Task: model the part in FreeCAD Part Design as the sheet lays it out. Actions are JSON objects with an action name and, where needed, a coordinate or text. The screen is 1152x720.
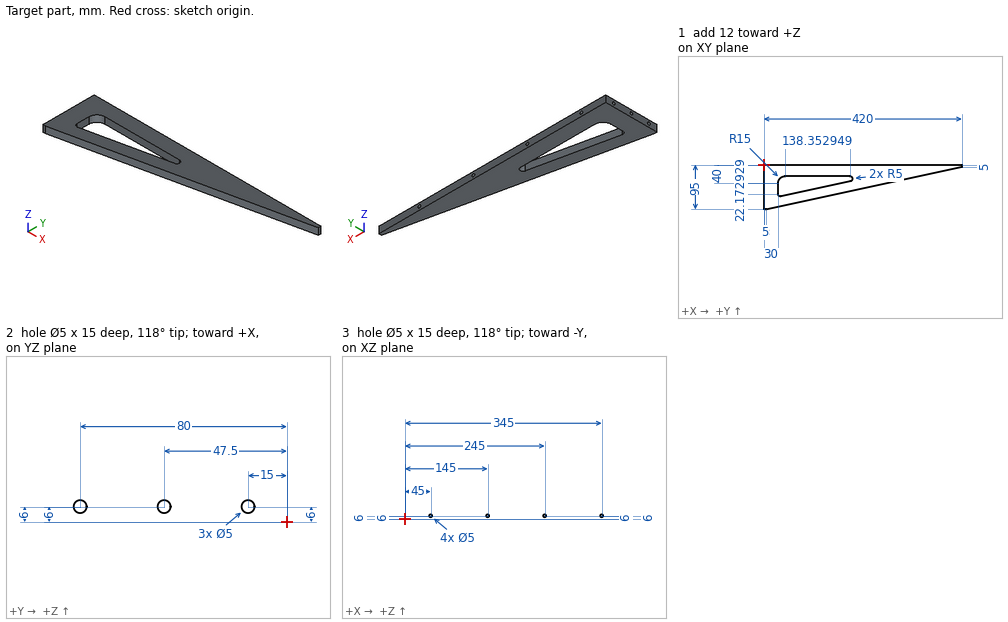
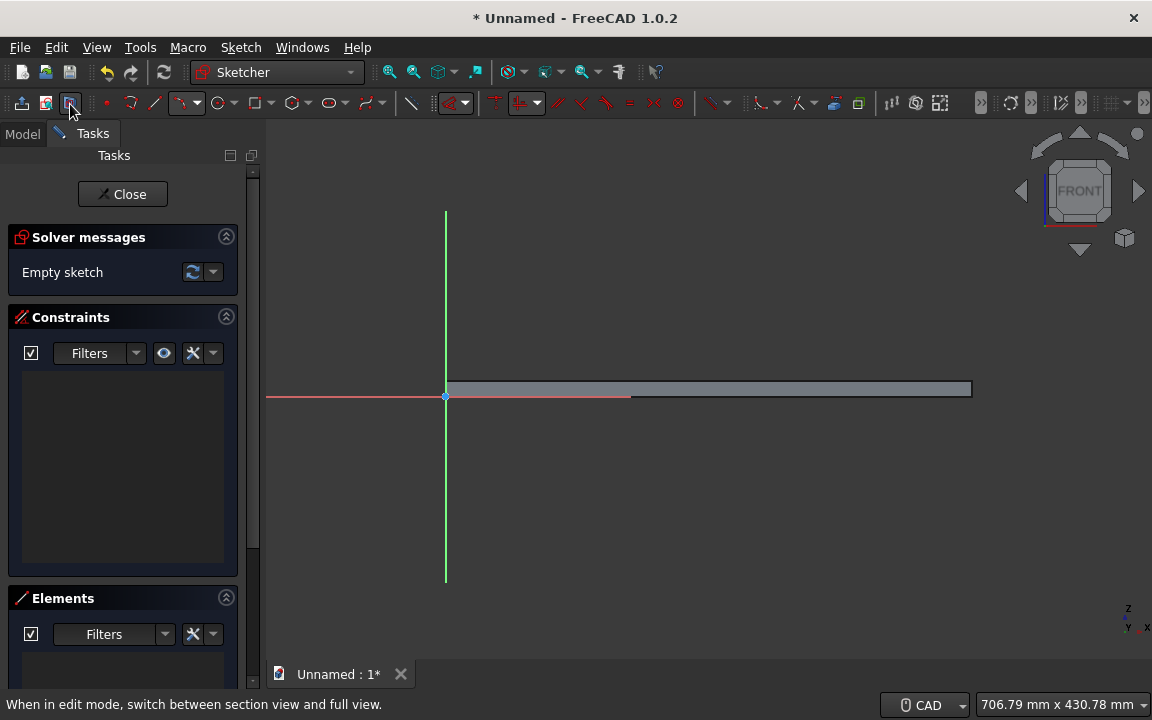
{"action": "left_click", "coordinate": [218, 104]}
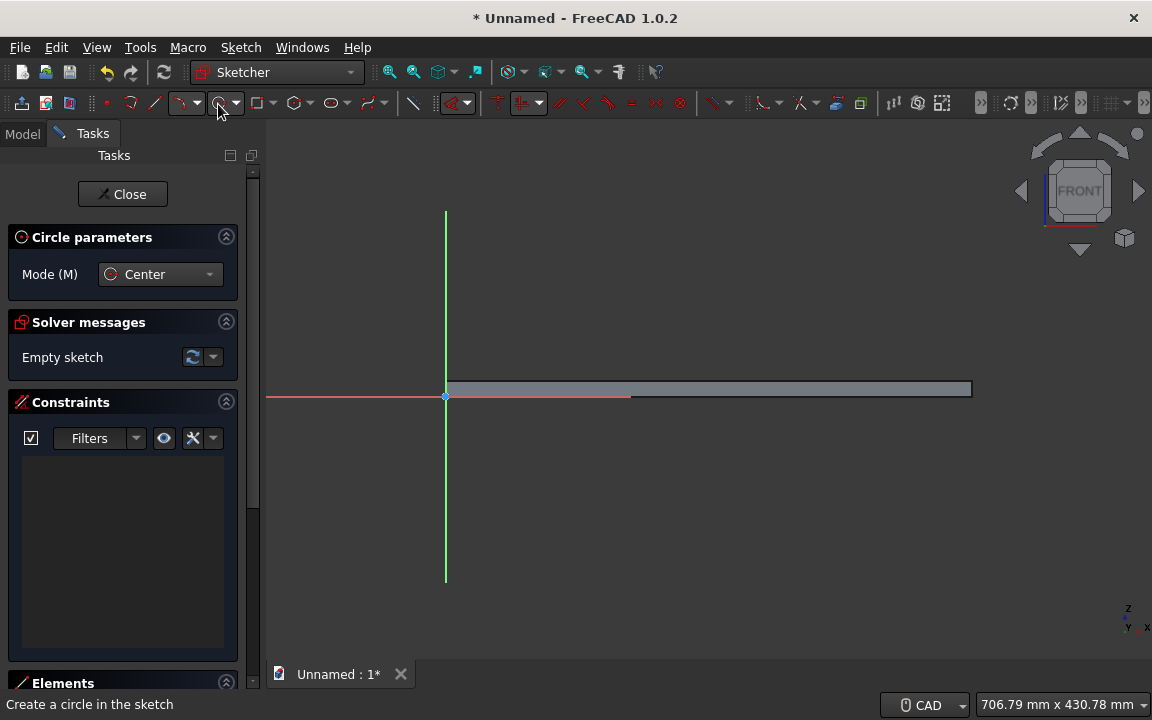
{"action": "scroll", "coordinate": [502, 389], "scroll_direction": "up", "scroll_amount": 10}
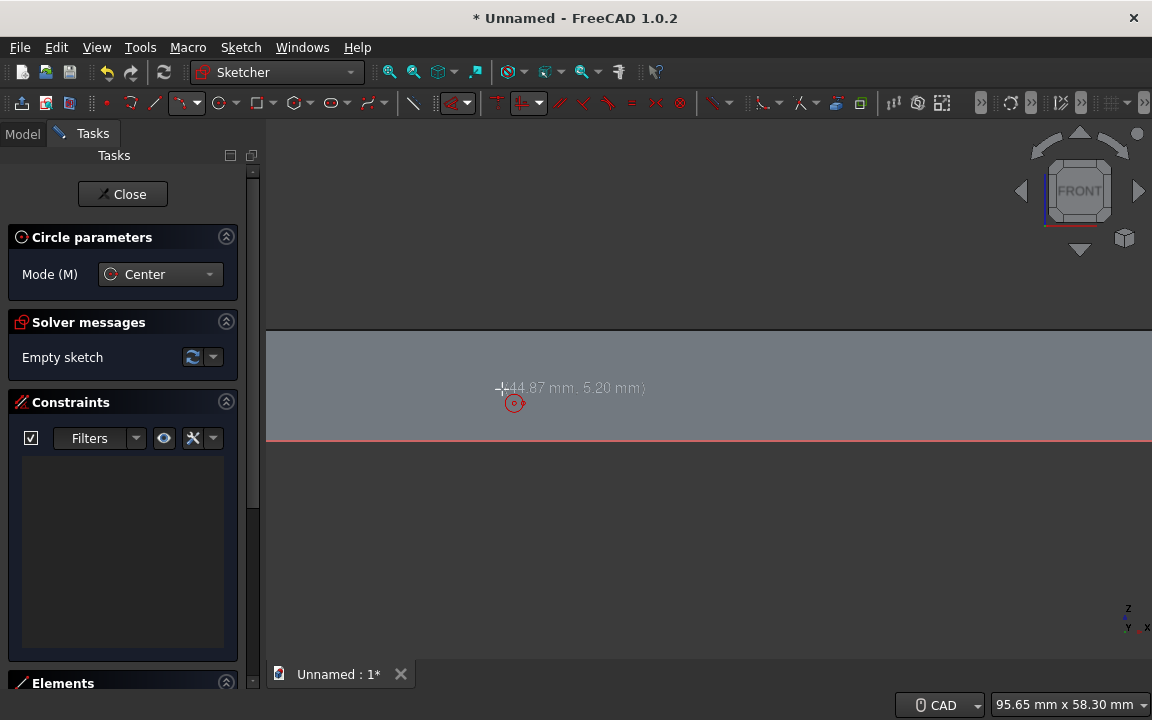
{"action": "scroll", "coordinate": [432, 386], "scroll_direction": "down", "scroll_amount": 9}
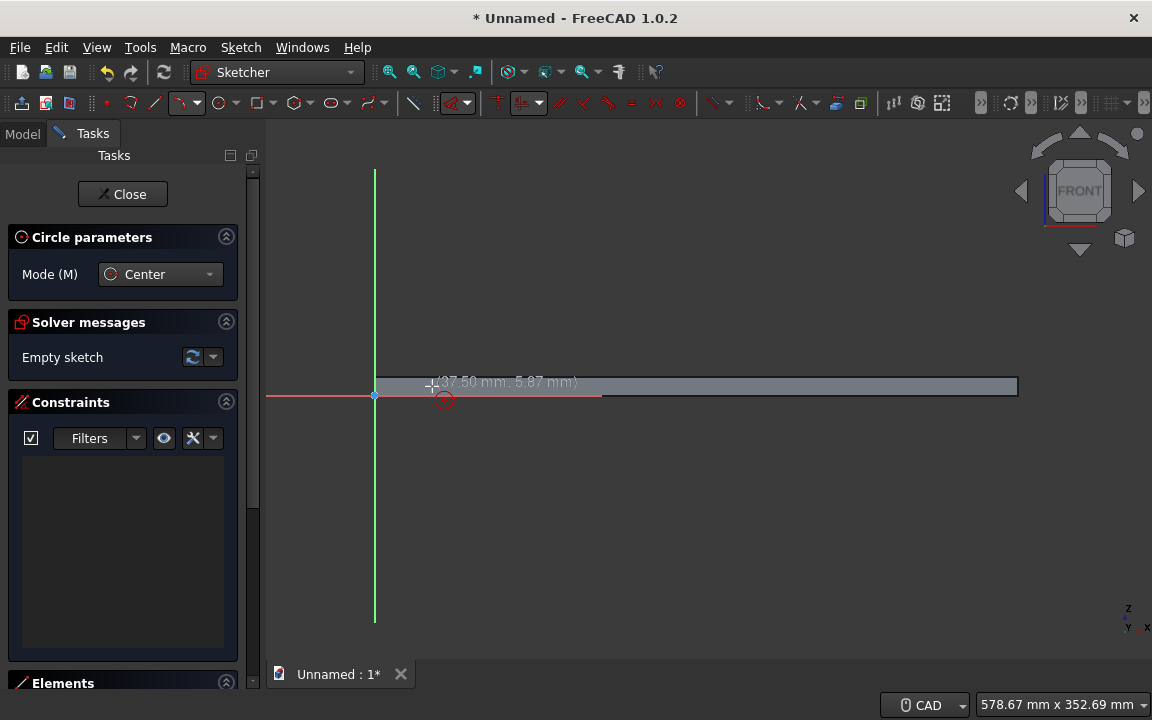
{"action": "scroll", "coordinate": [444, 386], "scroll_direction": "up", "scroll_amount": 3}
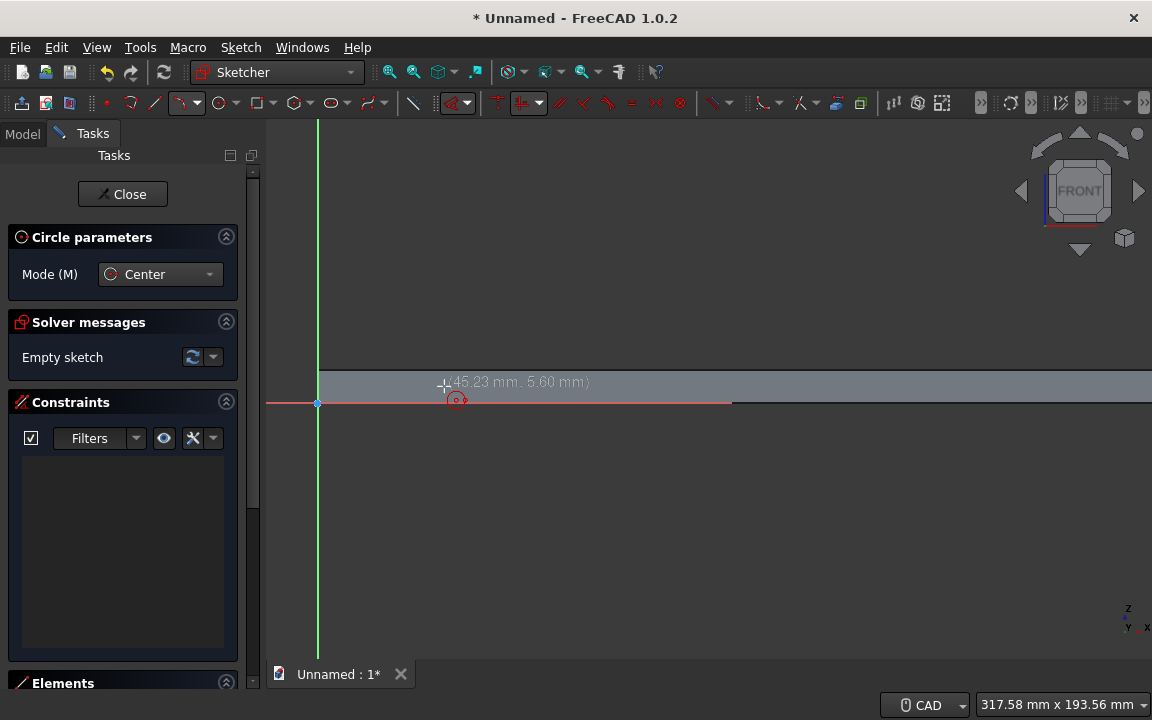
{"action": "left_click", "coordinate": [443, 386]}
{"action": "mouse_move", "coordinate": [448, 381]}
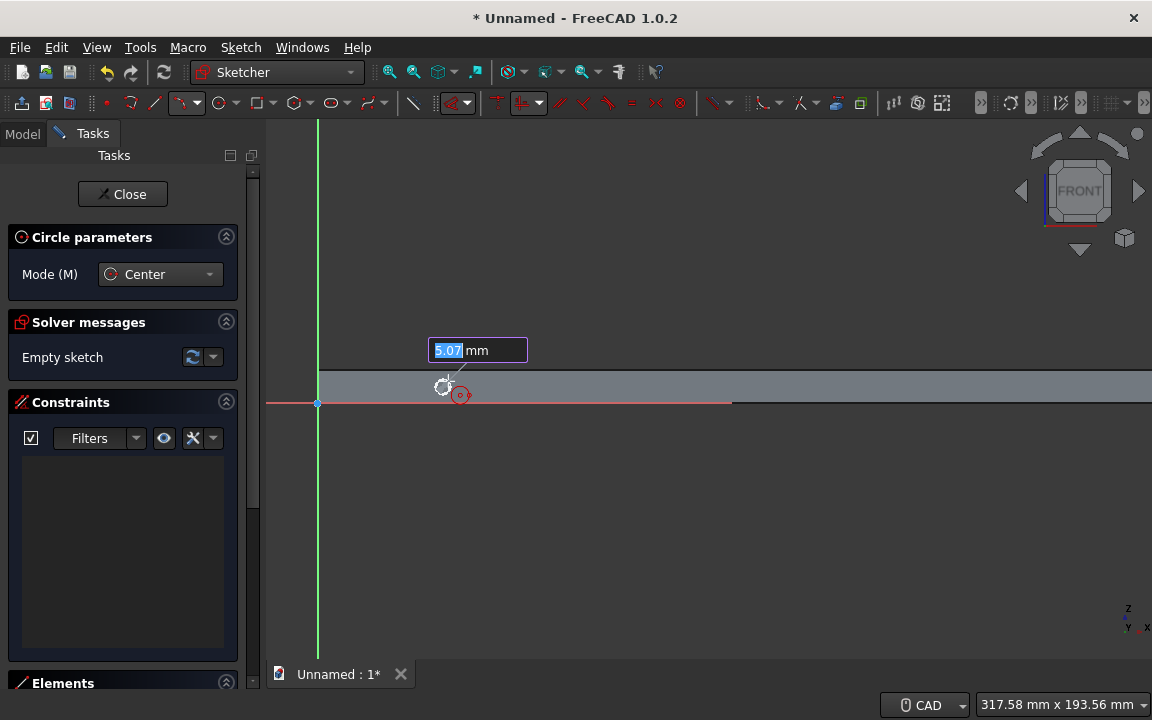
{"action": "type", "text": "5"}
{"action": "key", "text": "Return"}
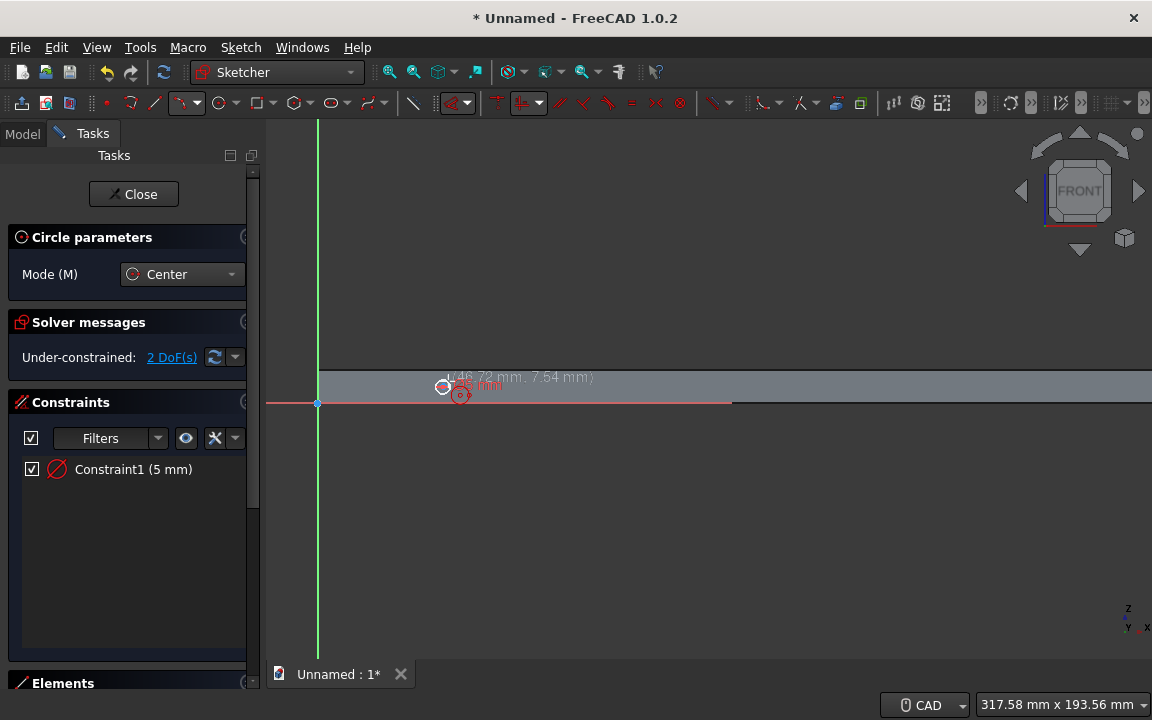
{"action": "scroll", "coordinate": [722, 386], "scroll_direction": "up", "scroll_amount": 6}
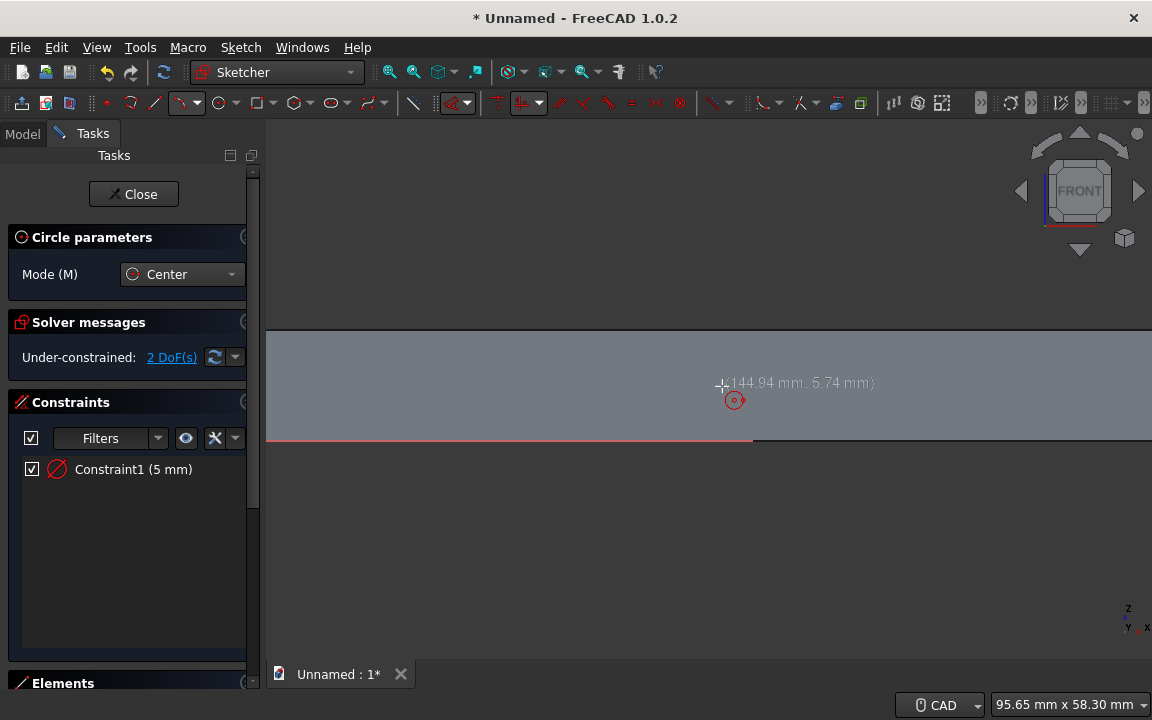
{"action": "scroll", "coordinate": [572, 386], "scroll_direction": "down", "scroll_amount": 9}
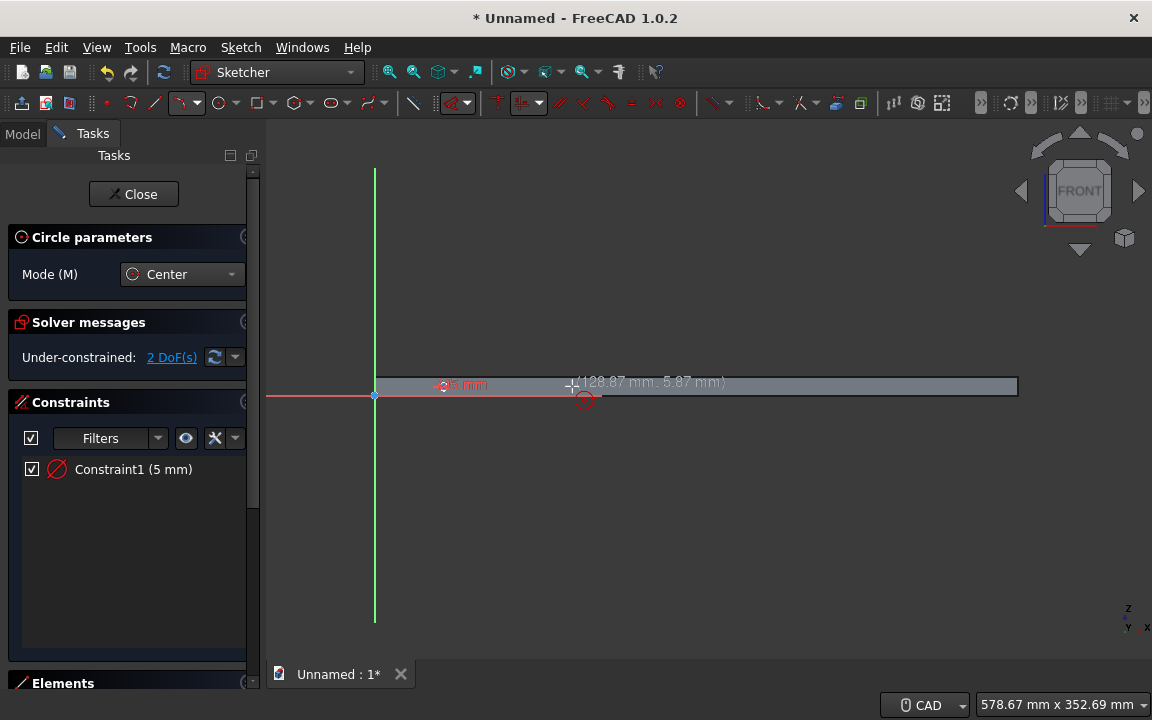
{"action": "scroll", "coordinate": [597, 386], "scroll_direction": "up", "scroll_amount": 3}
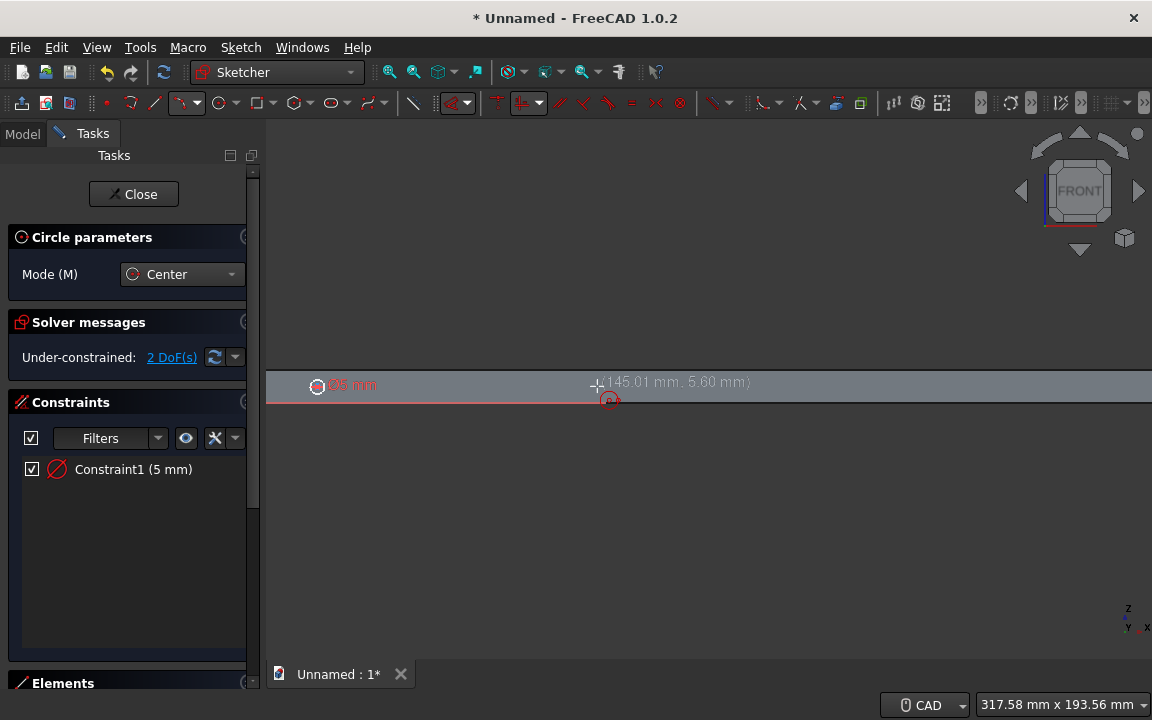
{"action": "left_click", "coordinate": [597, 386]}
{"action": "mouse_move", "coordinate": [602, 381]}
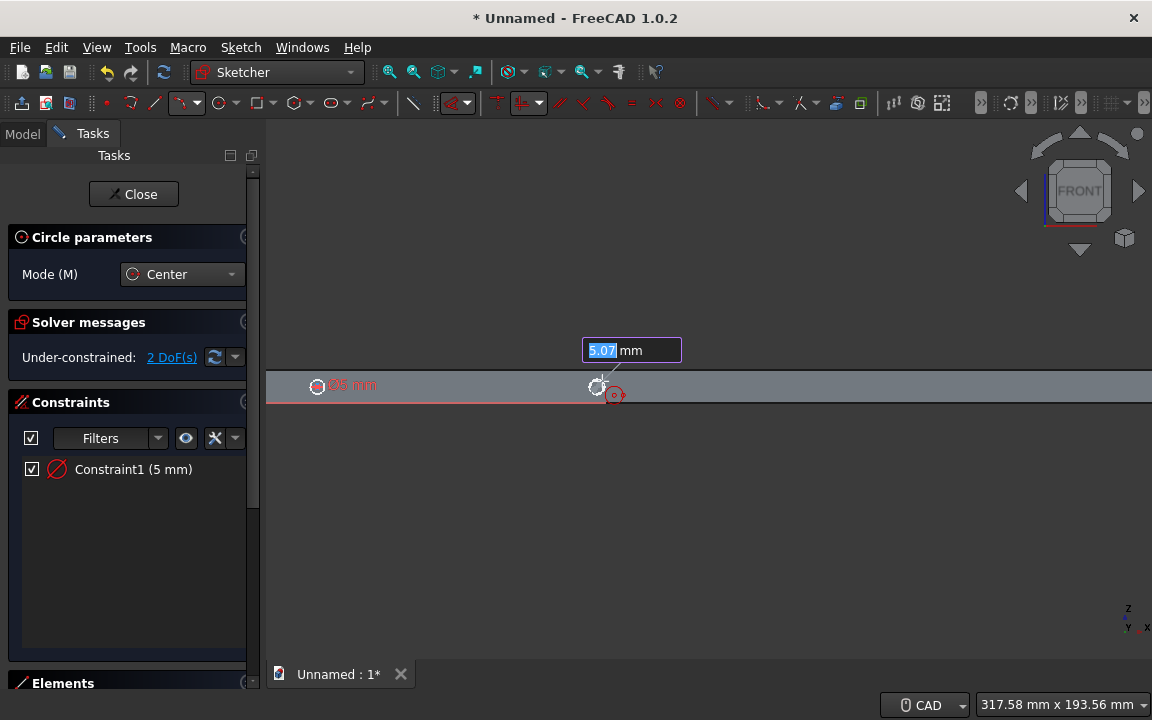
{"action": "type", "text": "5"}
{"action": "key", "text": "Return"}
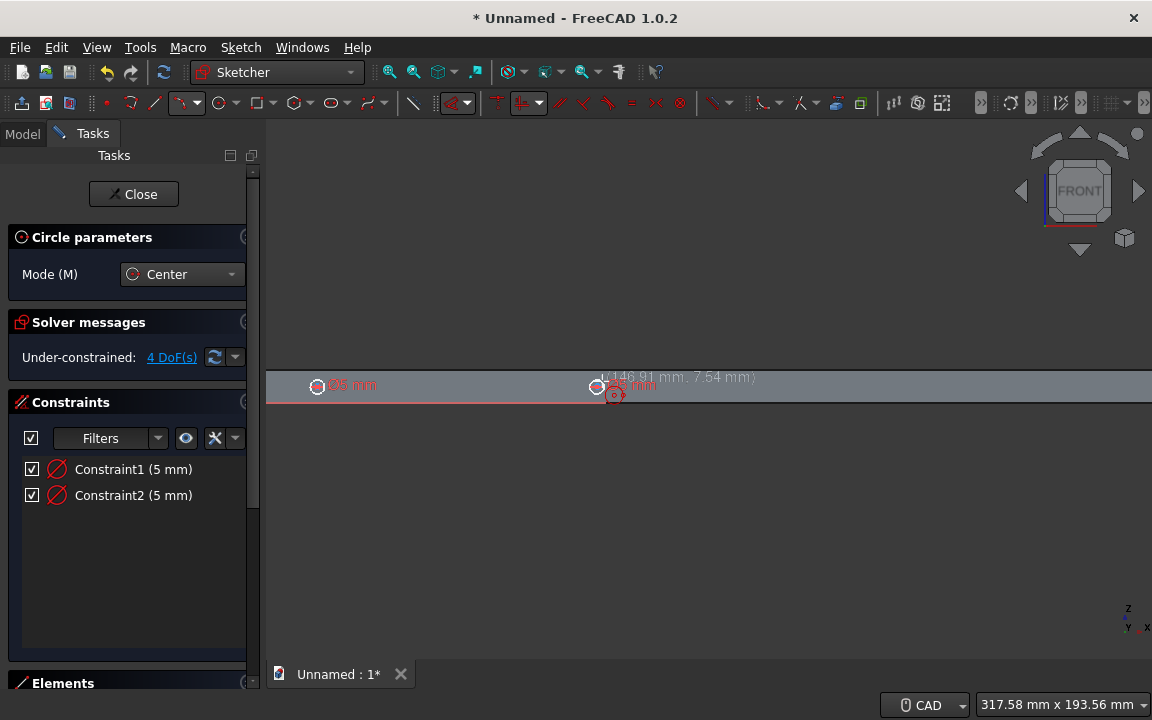
{"action": "scroll", "coordinate": [876, 386], "scroll_direction": "up", "scroll_amount": 6}